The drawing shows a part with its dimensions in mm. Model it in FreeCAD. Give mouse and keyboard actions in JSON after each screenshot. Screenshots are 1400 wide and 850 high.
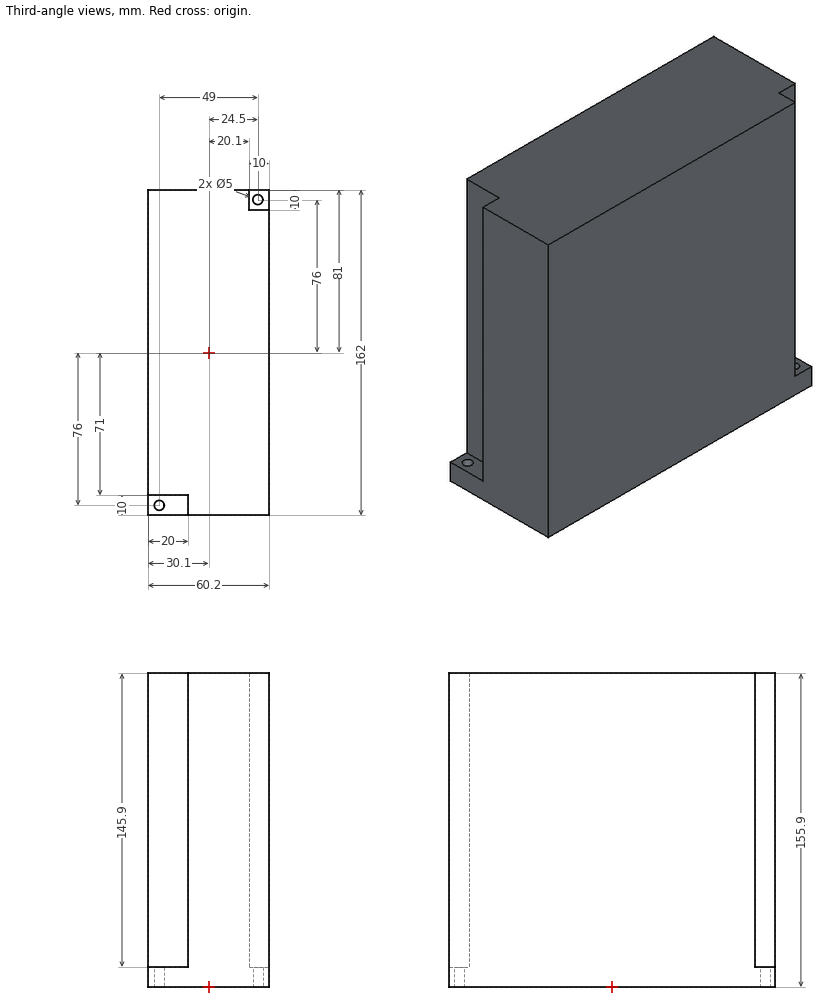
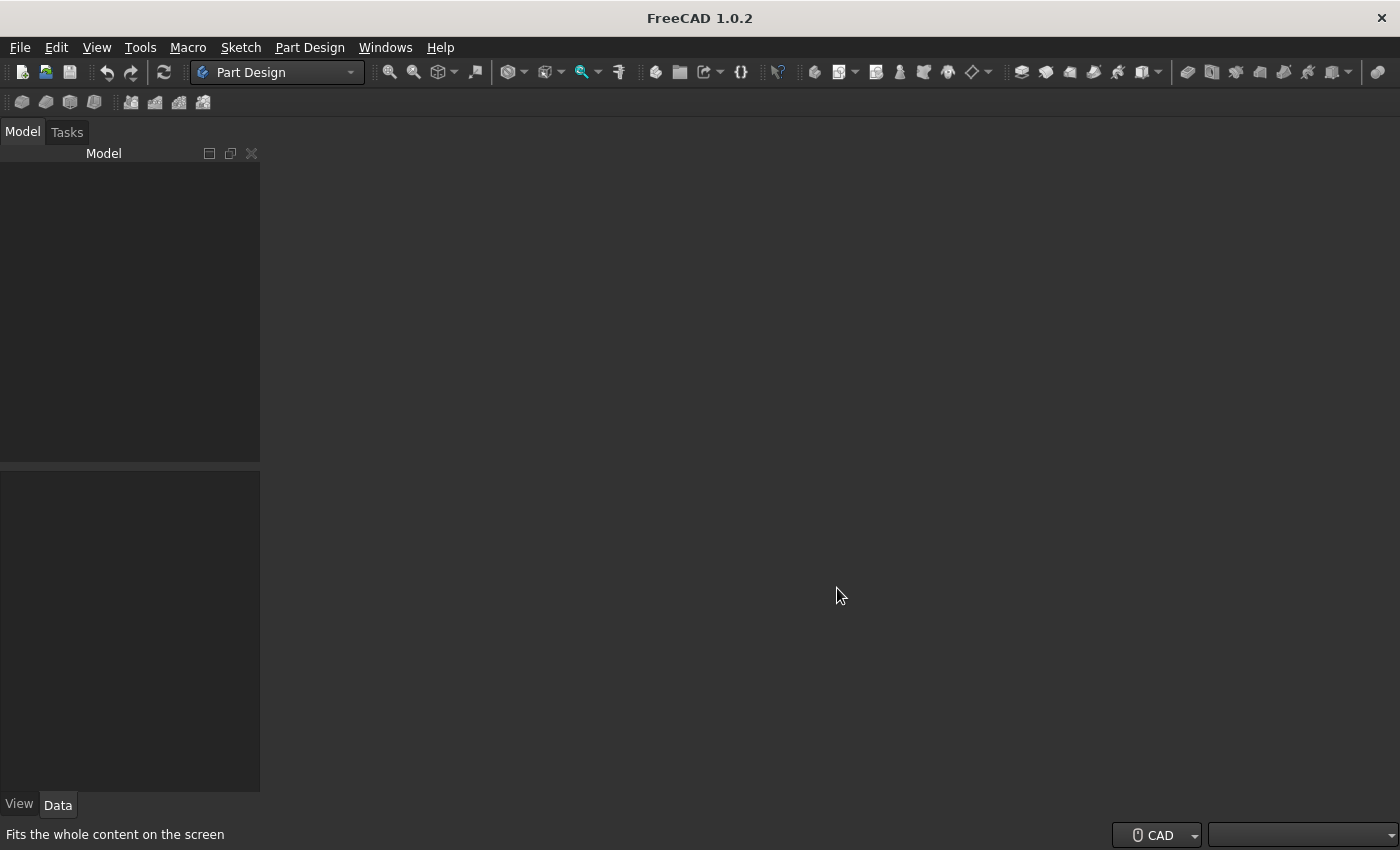
{"action": "left_click", "coordinate": [22, 72]}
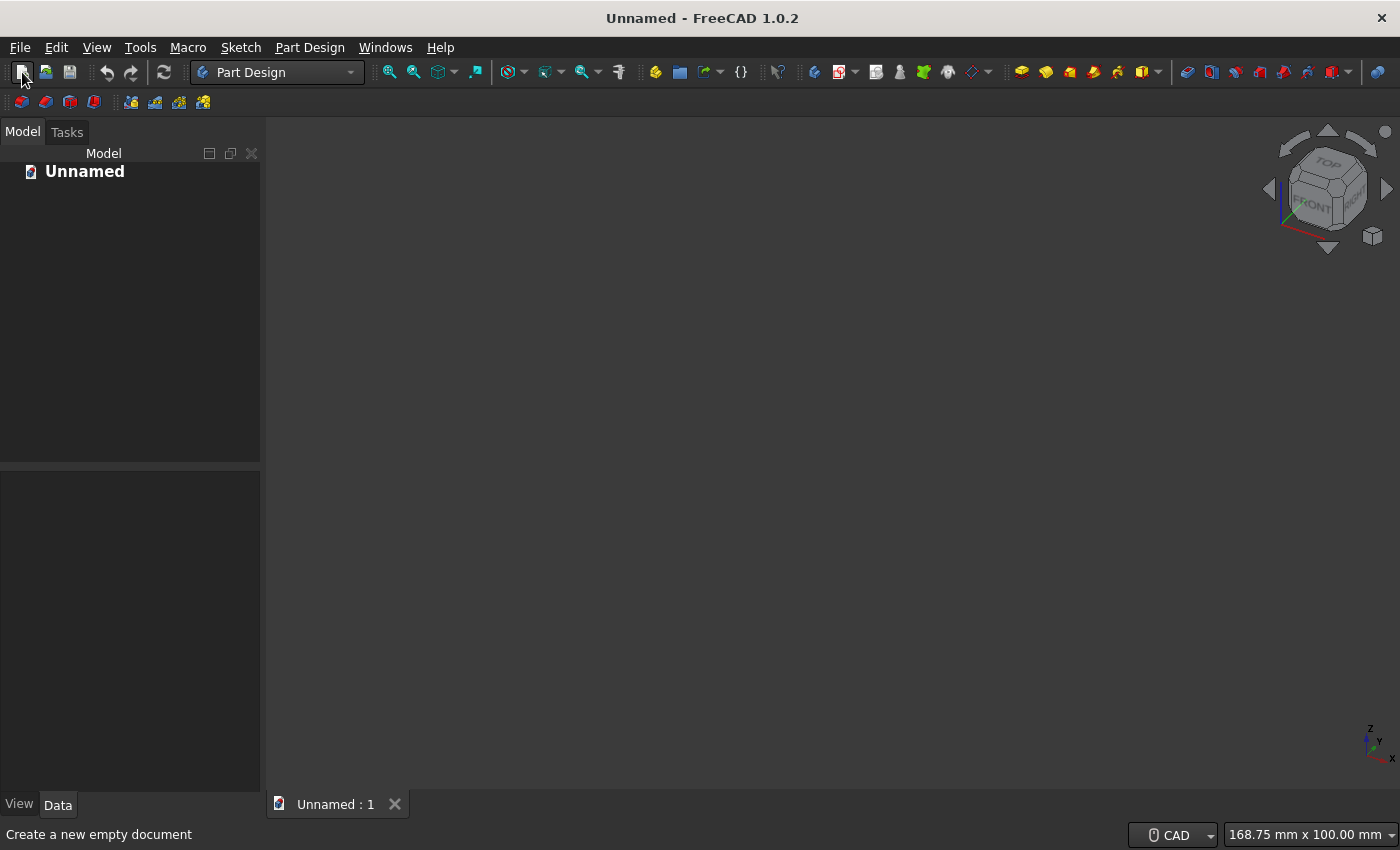
{"action": "left_click", "coordinate": [840, 72]}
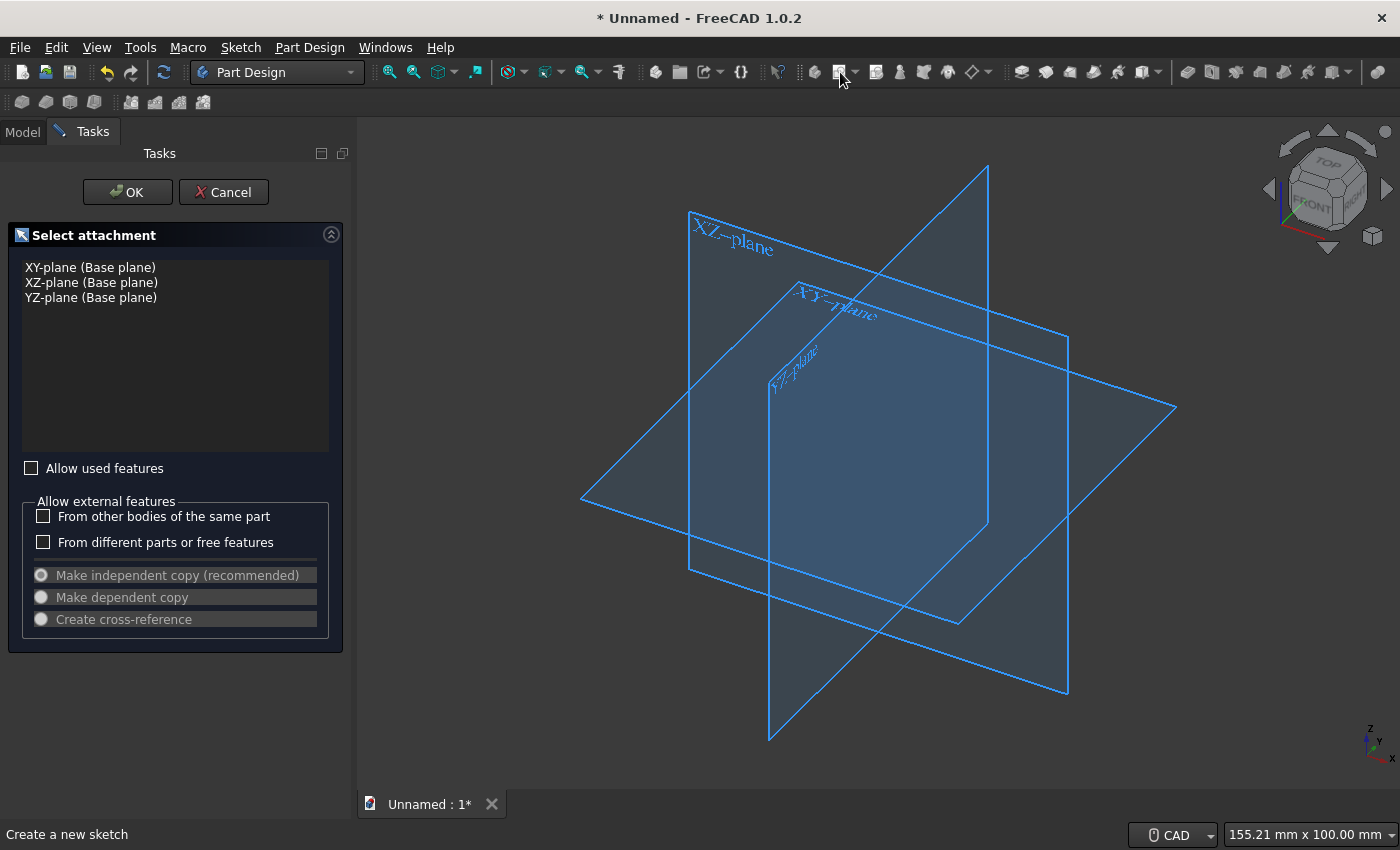
{"action": "left_click", "coordinate": [82, 268]}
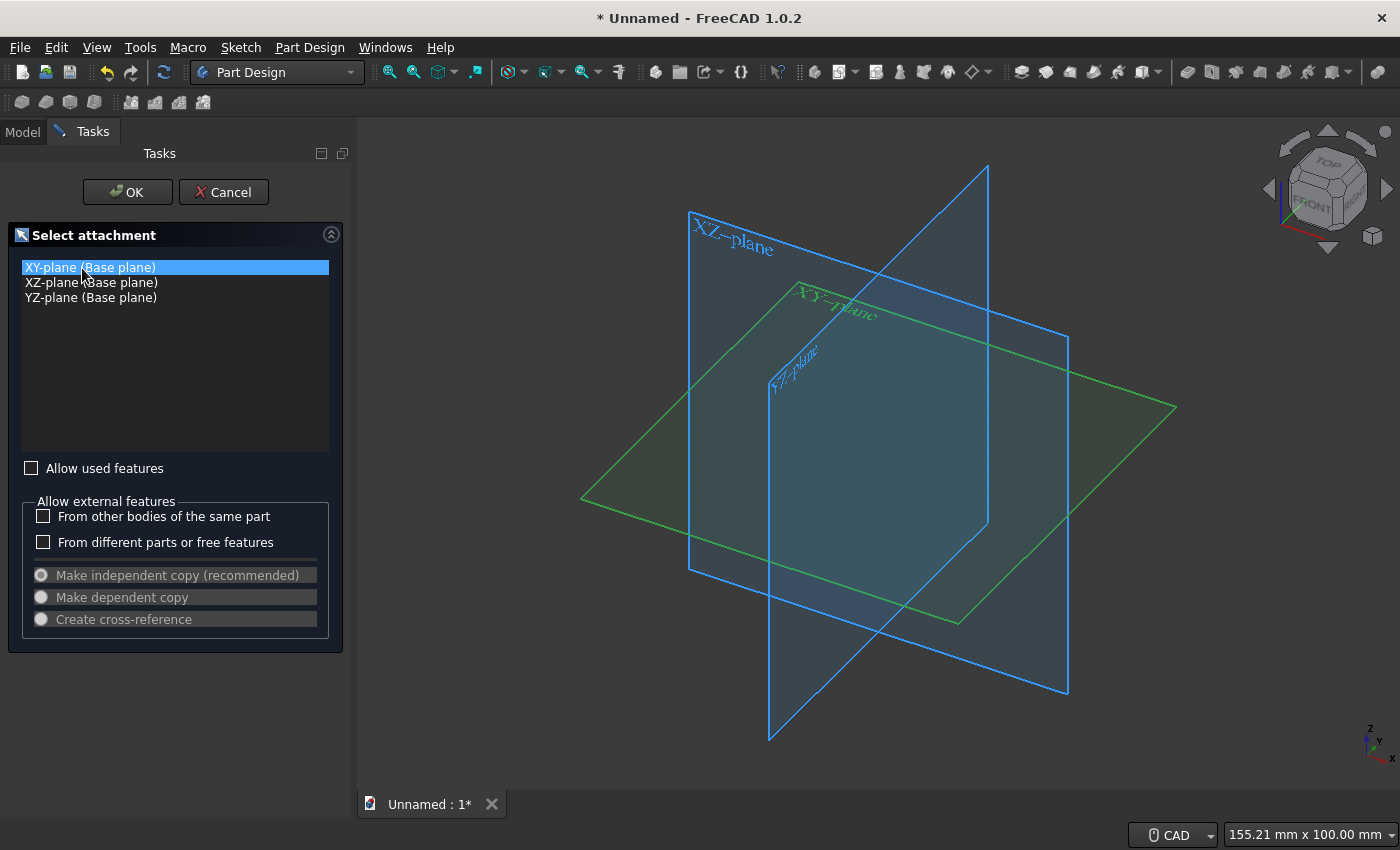
{"action": "left_click", "coordinate": [128, 192]}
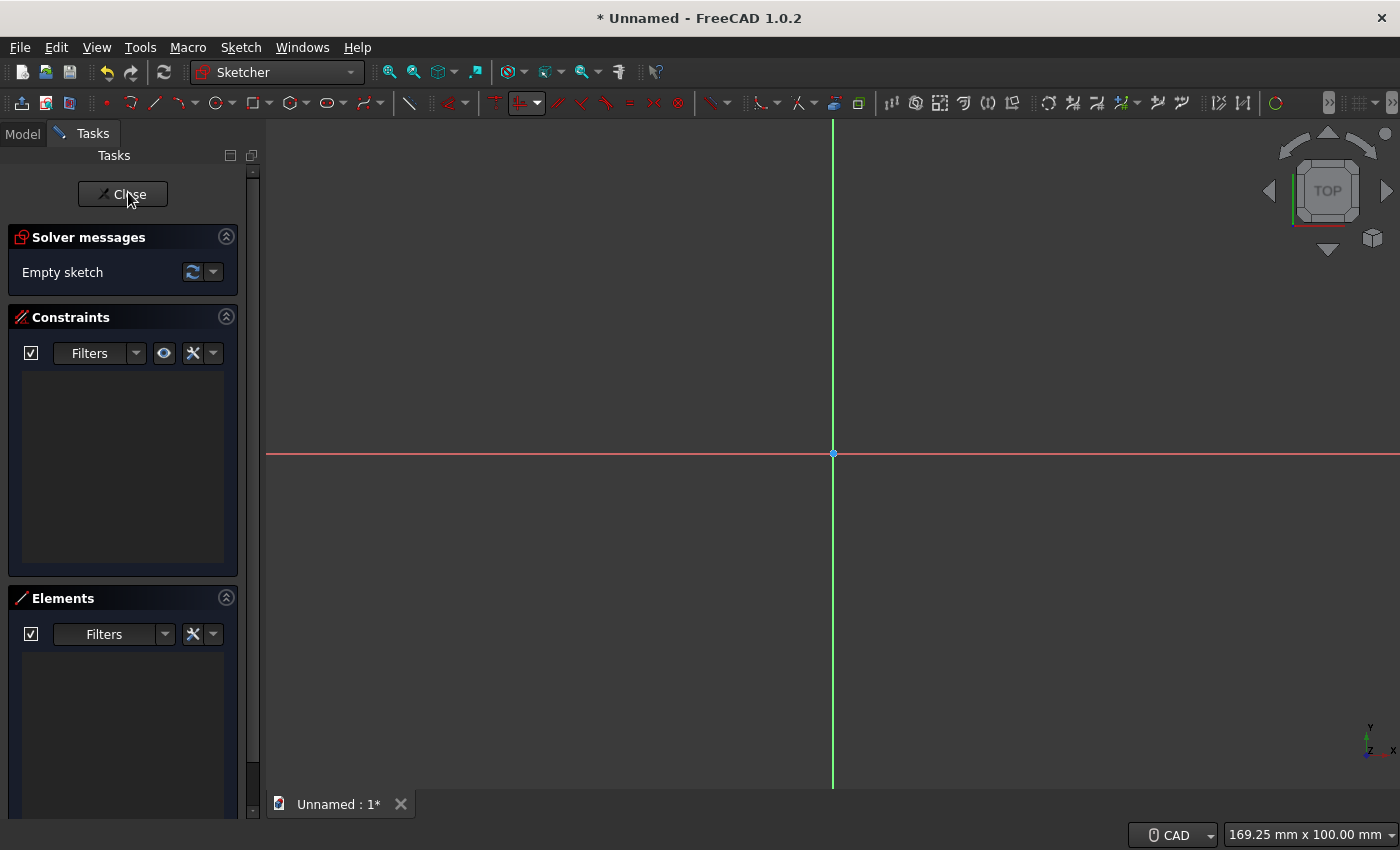
{"action": "scroll", "coordinate": [725, 454], "scroll_direction": "down", "scroll_amount": 5}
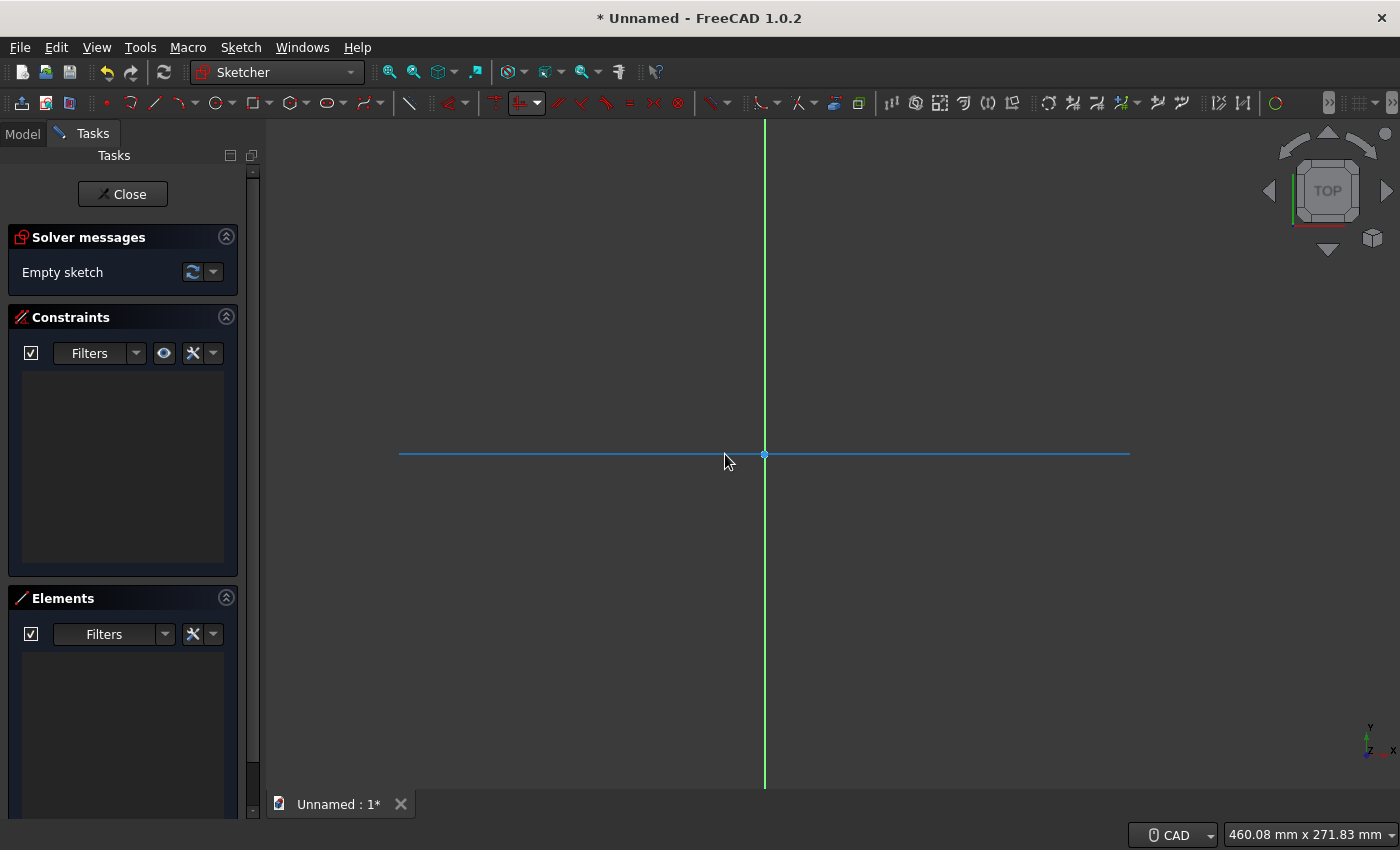
{"action": "left_click", "coordinate": [272, 104]}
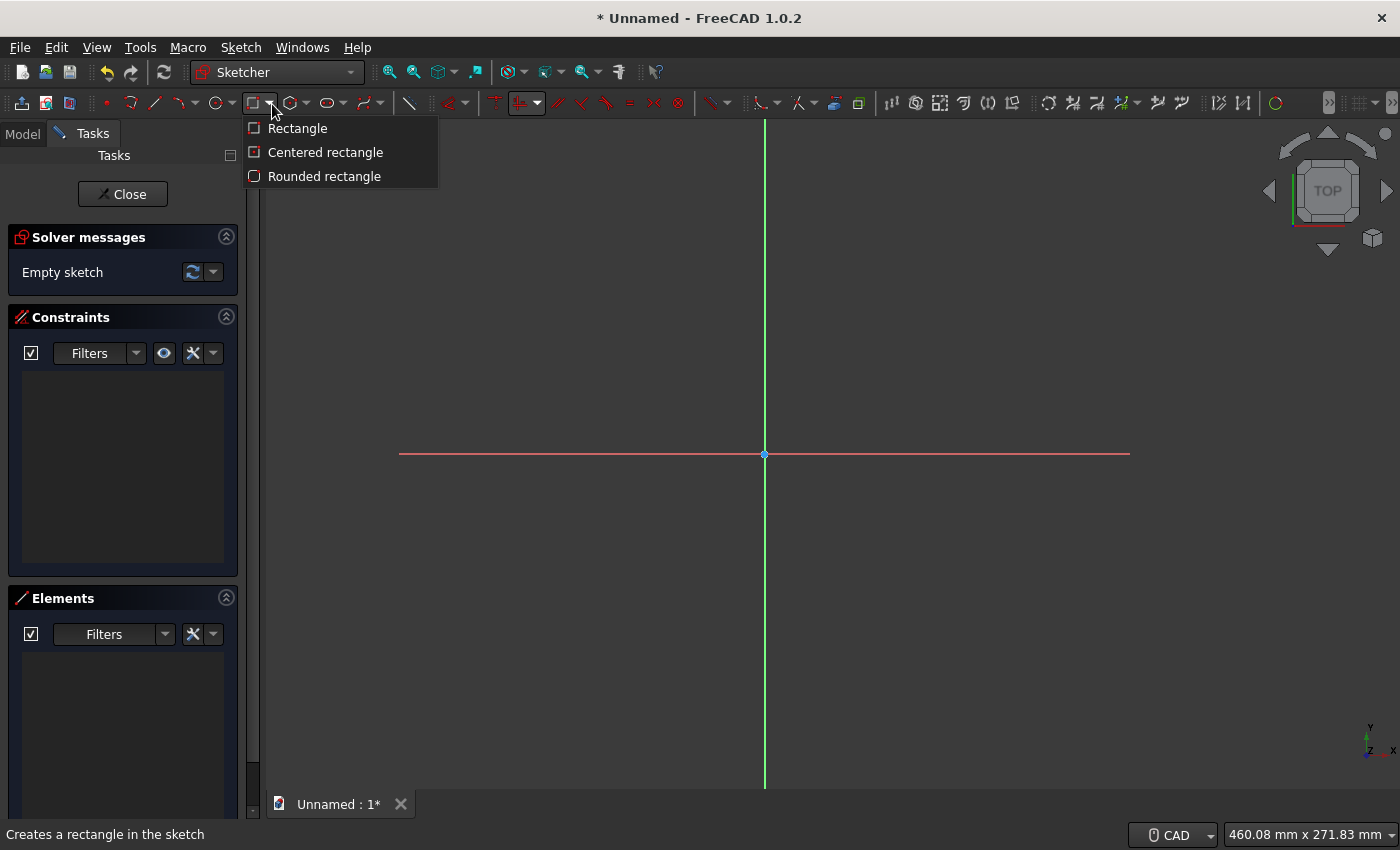
{"action": "left_click", "coordinate": [340, 152]}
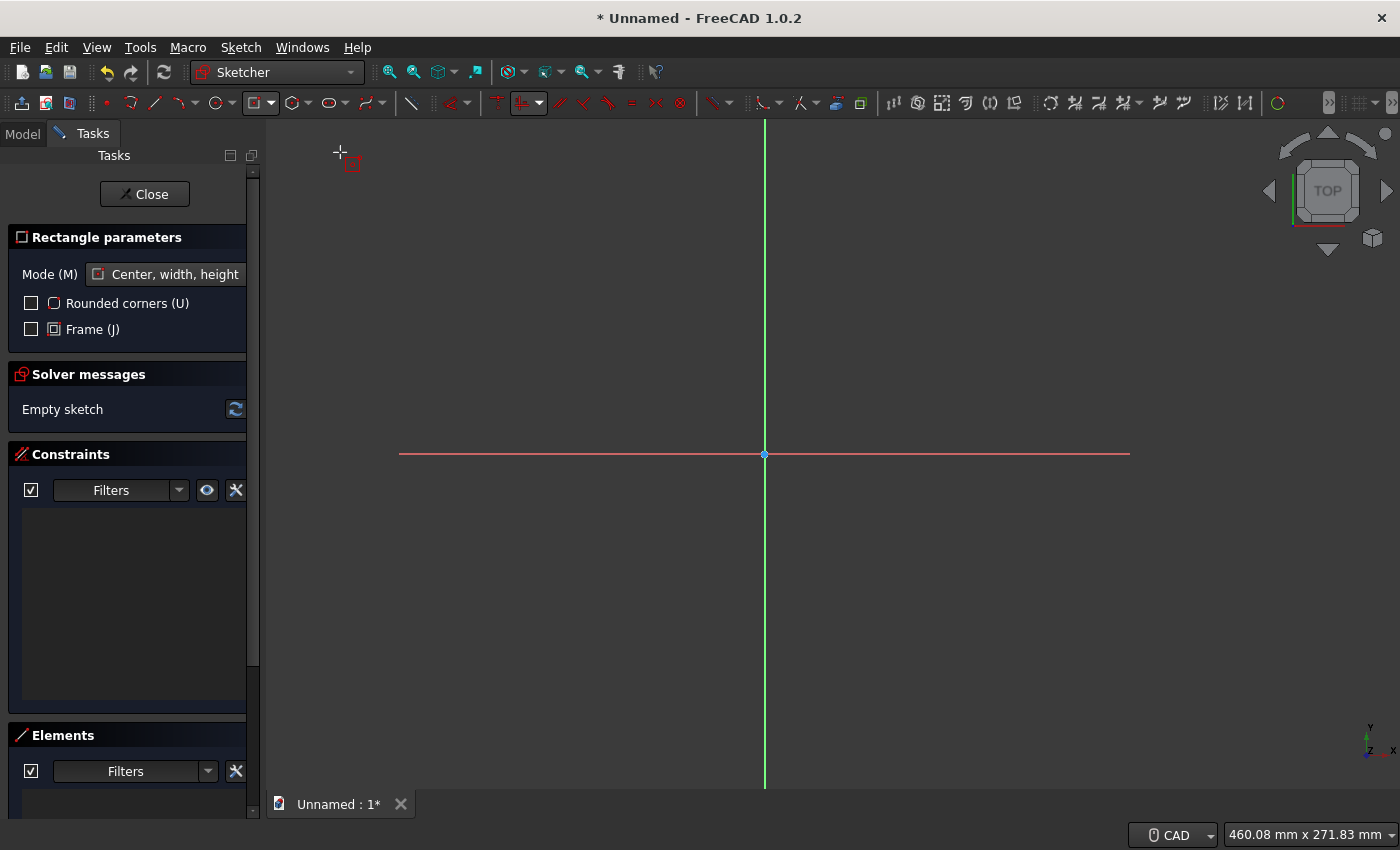
{"action": "left_click", "coordinate": [765, 454]}
{"action": "left_click", "coordinate": [839, 255]}
{"action": "key", "text": "Escape"}